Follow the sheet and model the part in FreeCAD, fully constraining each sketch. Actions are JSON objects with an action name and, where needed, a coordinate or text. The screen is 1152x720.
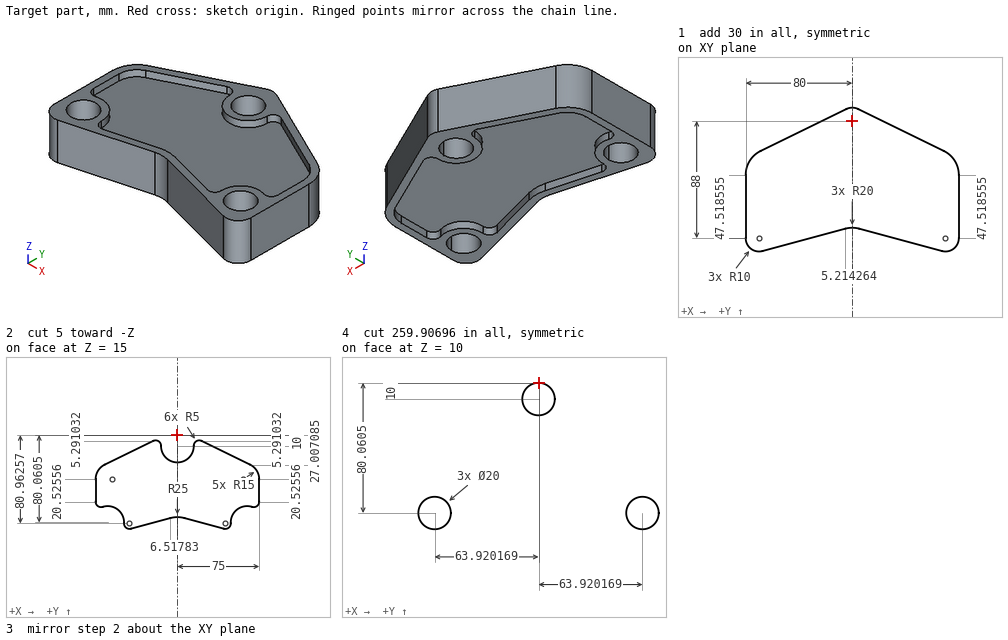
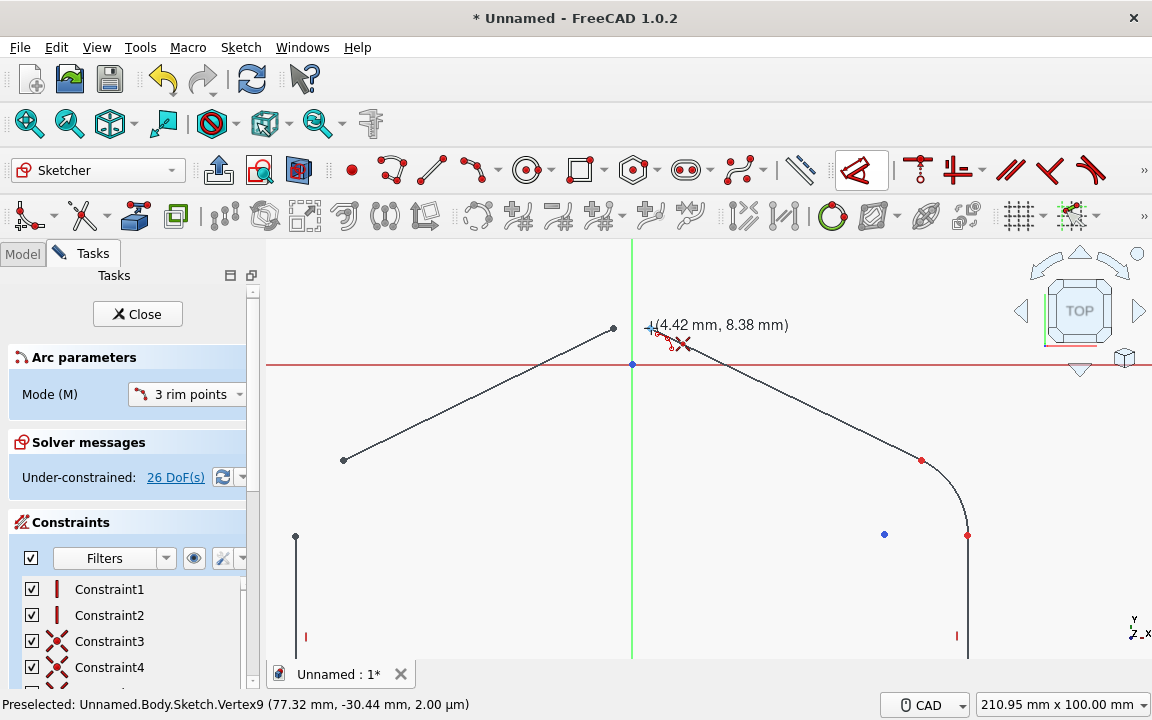
{"action": "left_click", "coordinate": [650, 329]}
{"action": "left_click", "coordinate": [613, 329]}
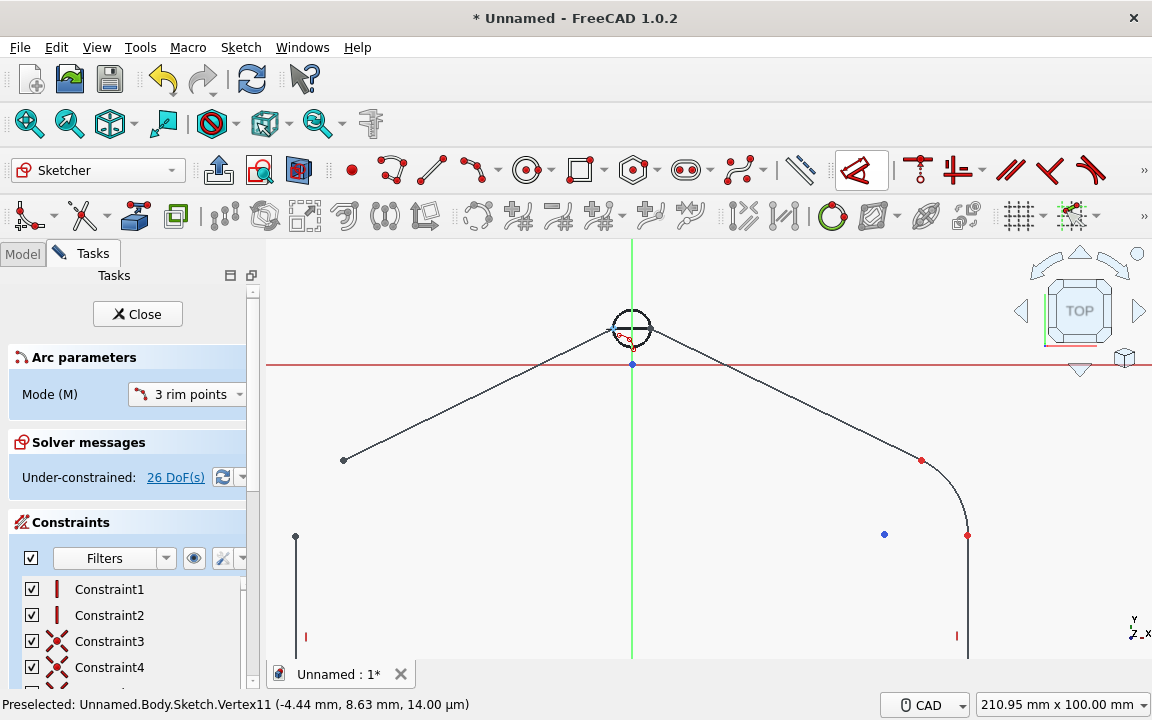
{"action": "scroll", "coordinate": [636, 323], "scroll_direction": "up", "scroll_amount": 8}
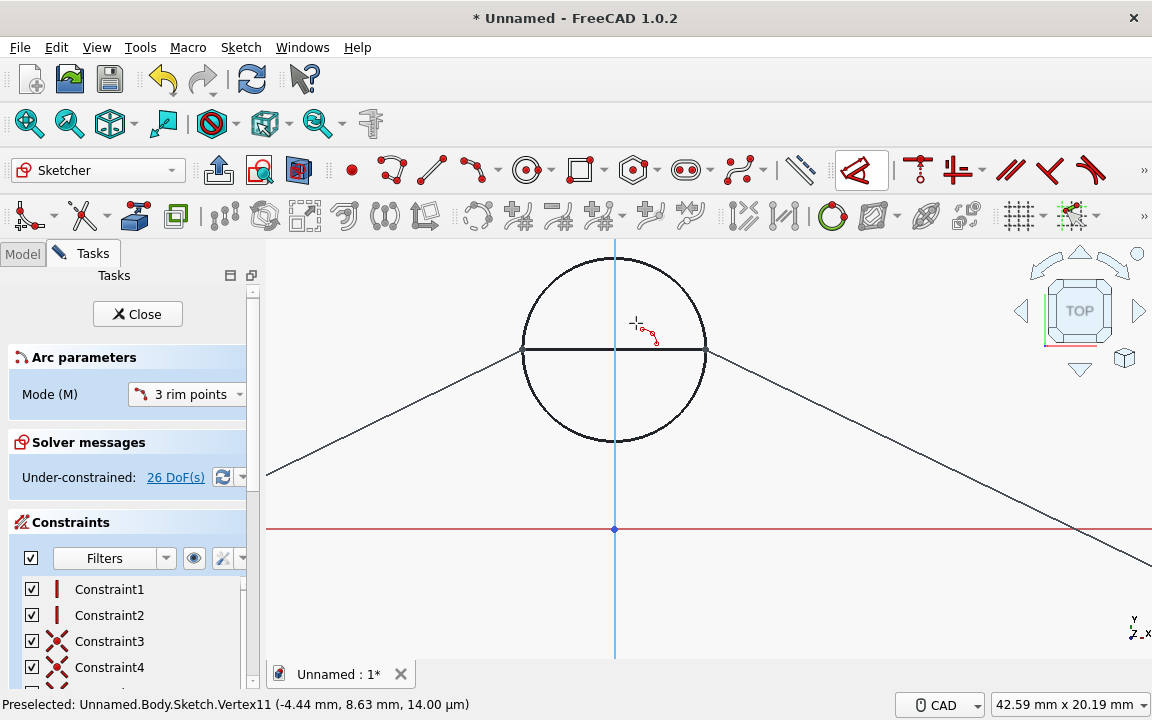
{"action": "left_click", "coordinate": [634, 322]}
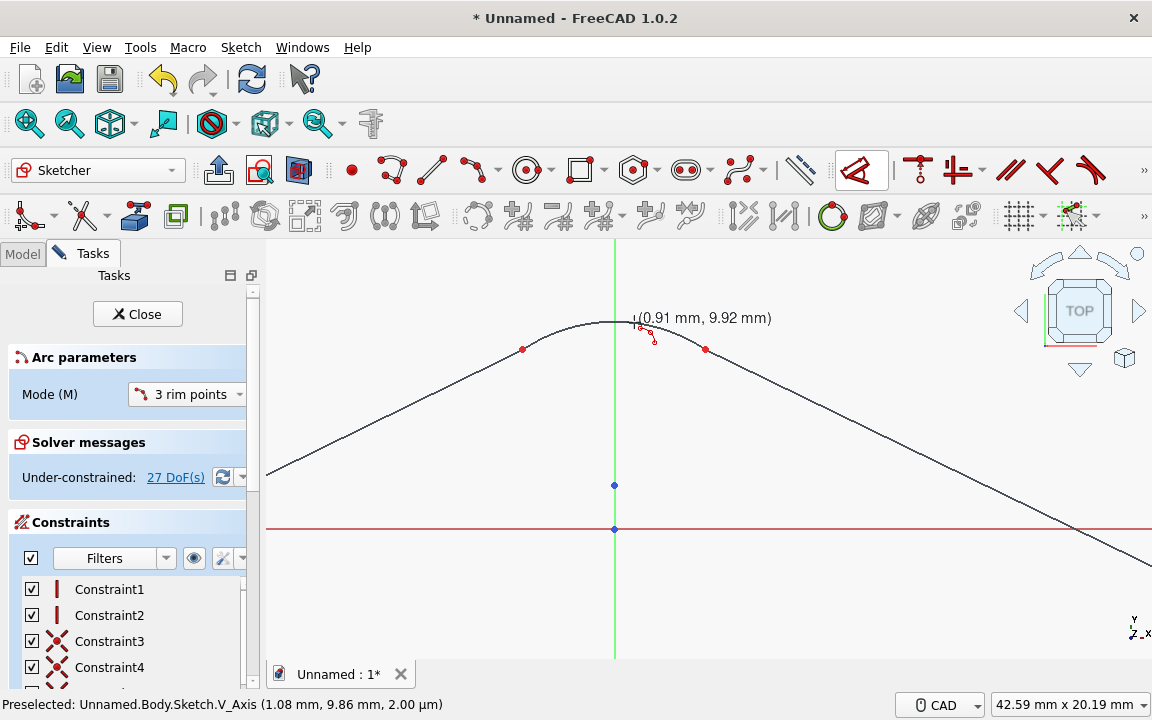
{"action": "scroll", "coordinate": [644, 325], "scroll_direction": "down", "scroll_amount": 11}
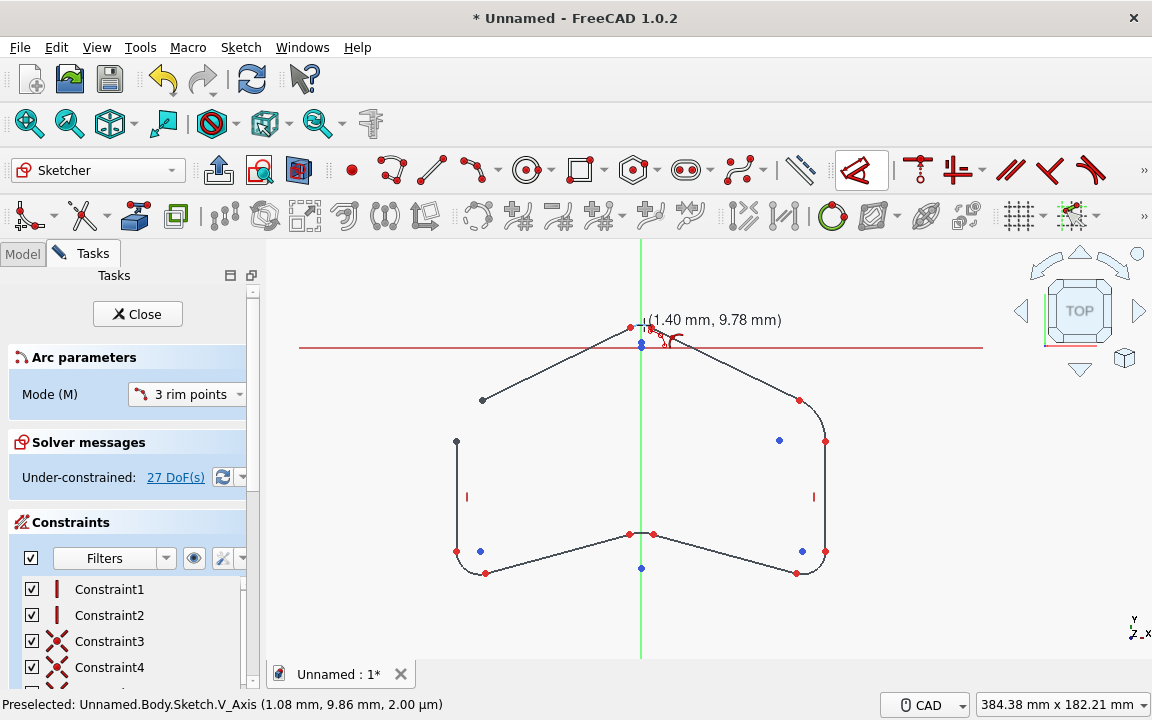
{"action": "left_click", "coordinate": [483, 400]}
{"action": "left_click", "coordinate": [457, 442]}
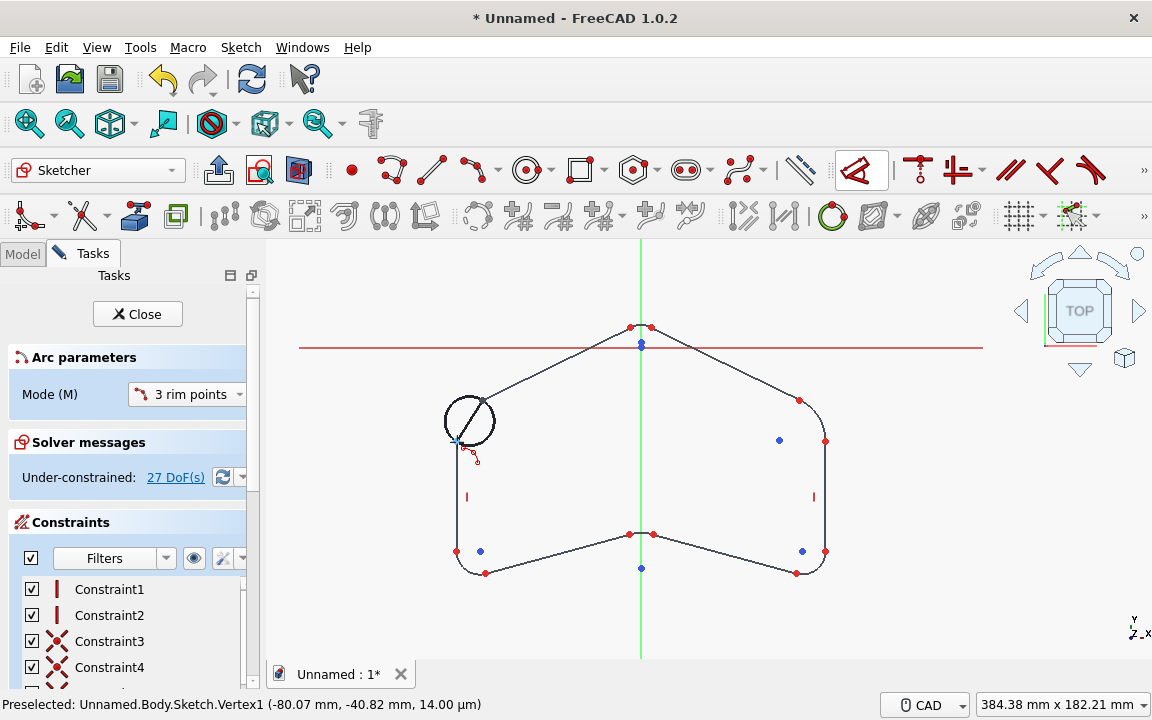
{"action": "scroll", "coordinate": [464, 417], "scroll_direction": "up", "scroll_amount": 5}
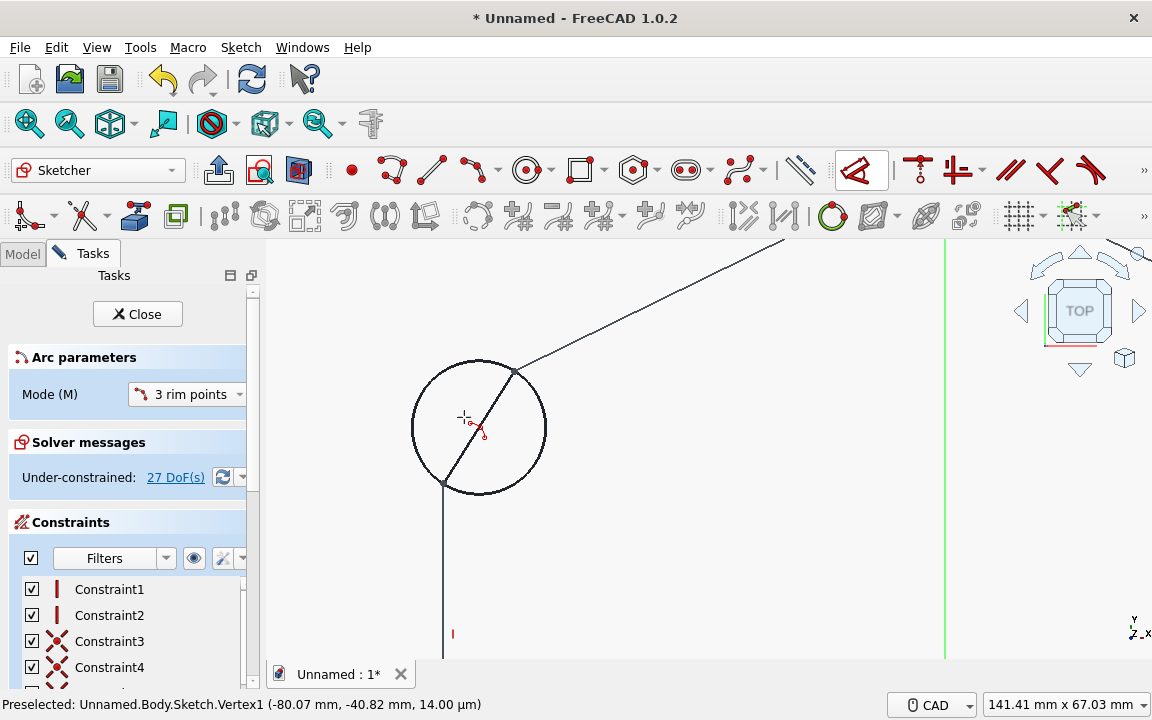
{"action": "left_click", "coordinate": [463, 416]}
{"action": "key", "text": "Escape"}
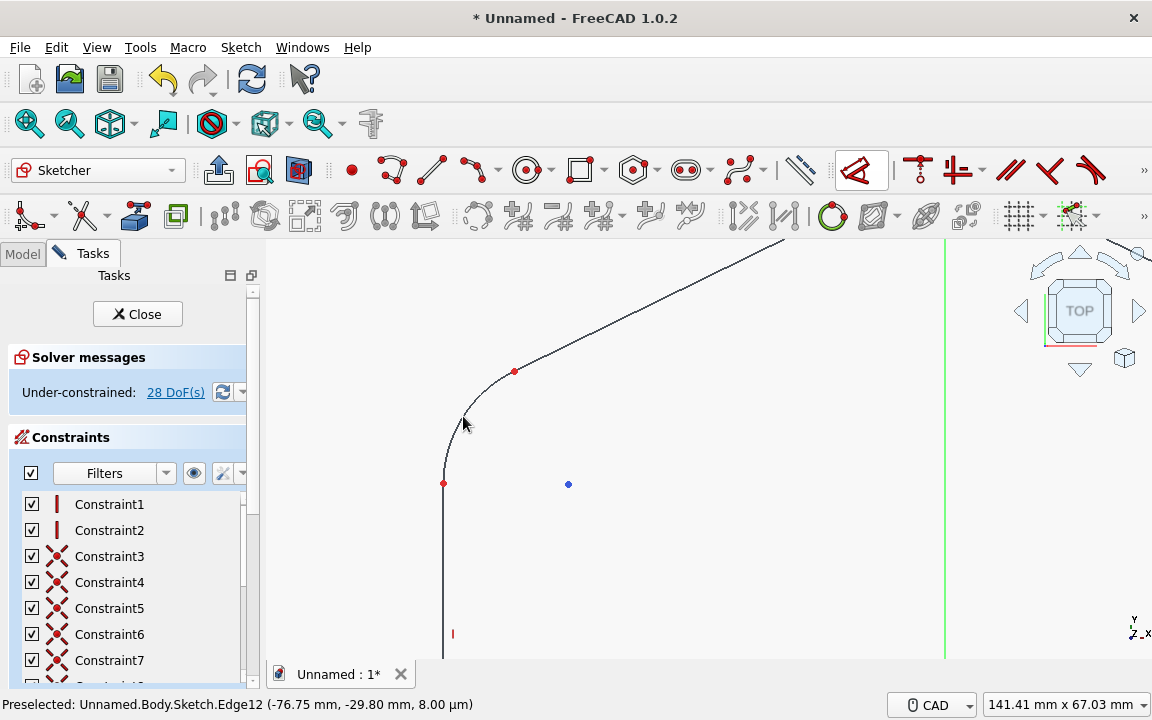
{"action": "left_click", "coordinate": [443, 574]}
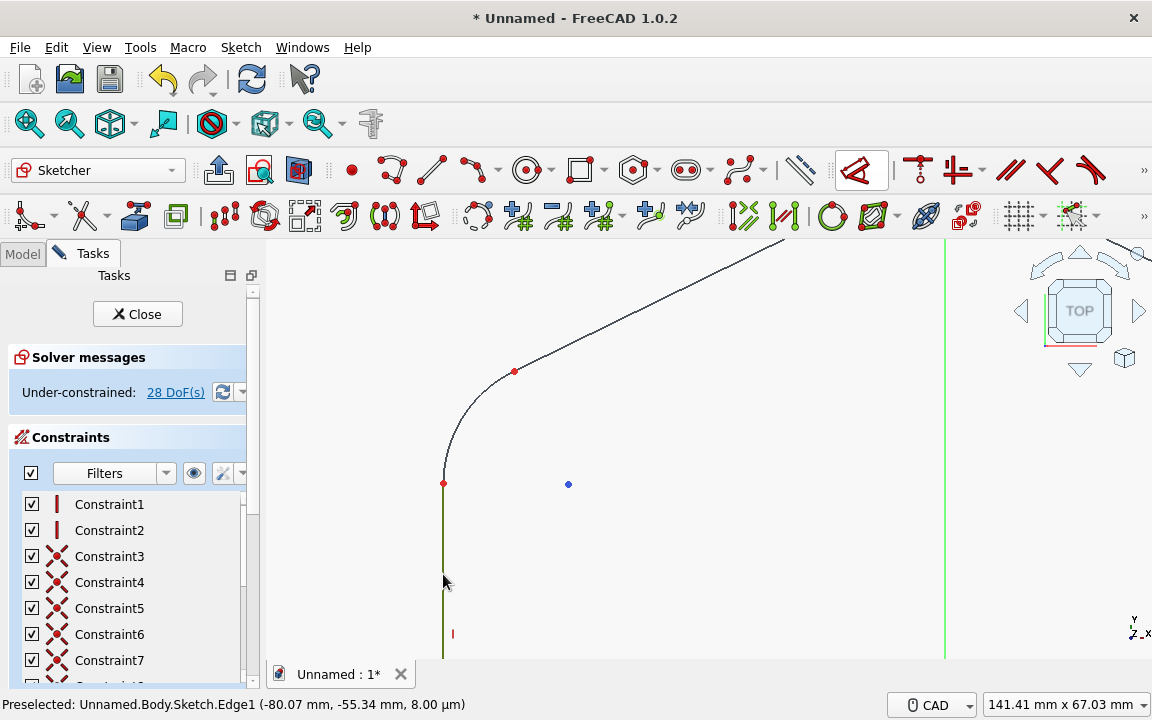
{"action": "scroll", "coordinate": [463, 418], "scroll_direction": "down", "scroll_amount": 5}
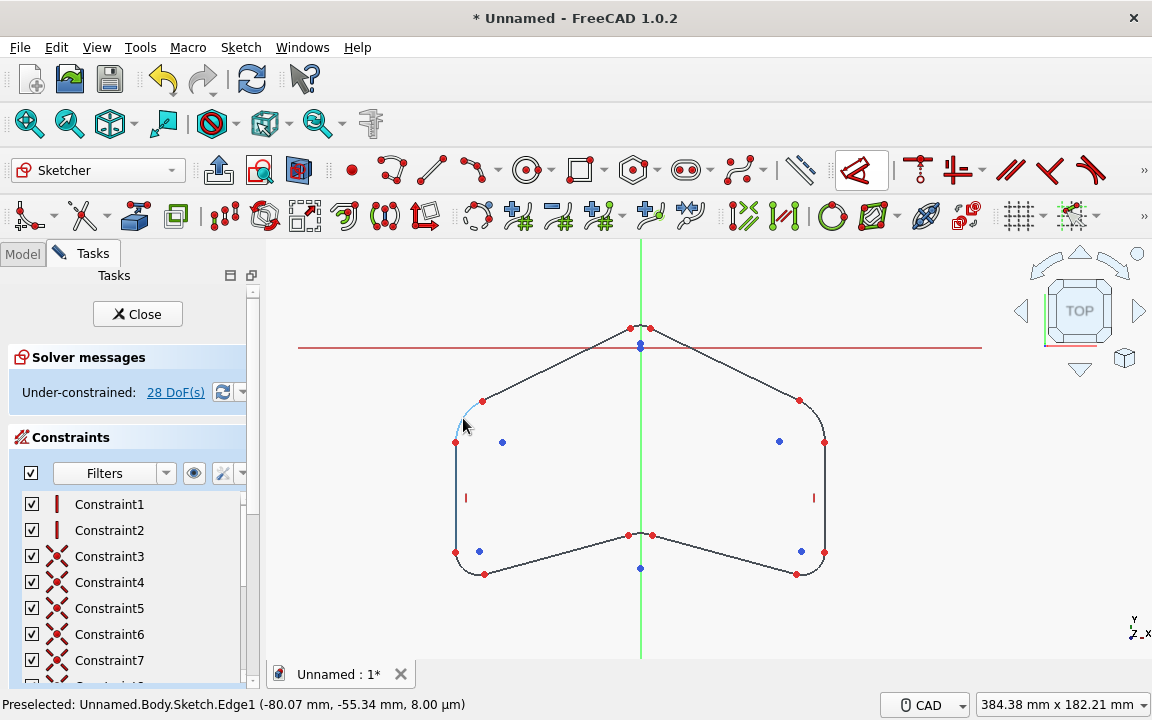
{"action": "left_click", "coordinate": [460, 564]}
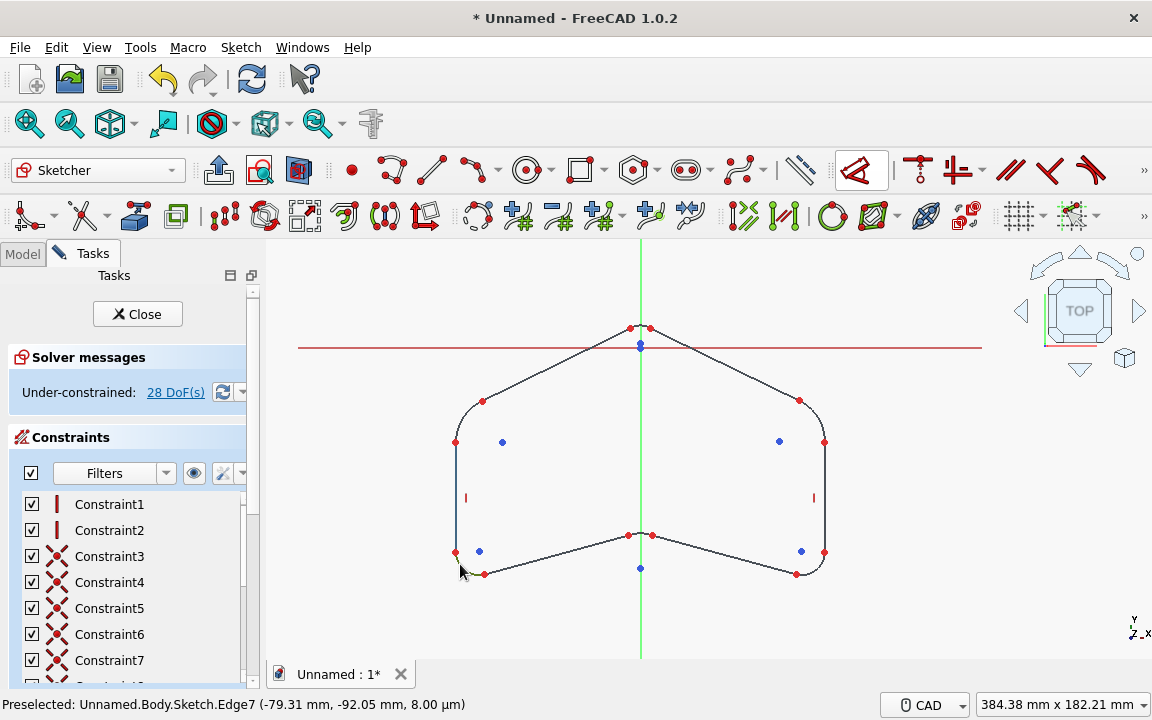
{"action": "left_click", "coordinate": [1092, 170]}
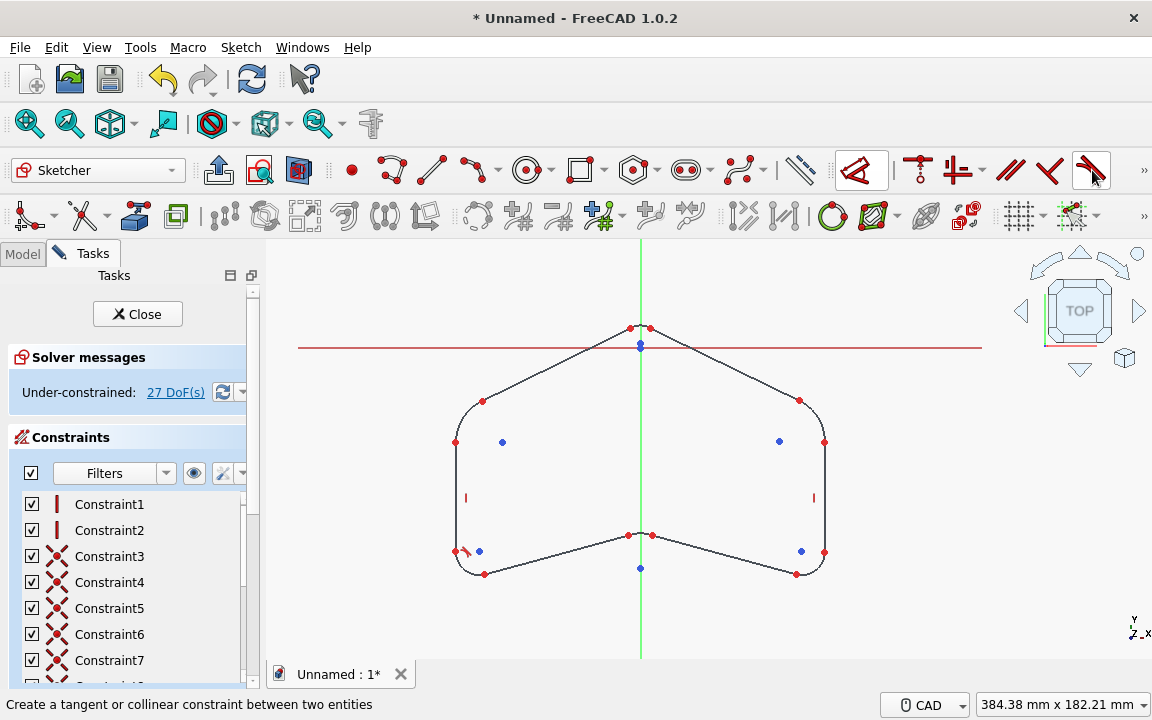
{"action": "left_click", "coordinate": [456, 475]}